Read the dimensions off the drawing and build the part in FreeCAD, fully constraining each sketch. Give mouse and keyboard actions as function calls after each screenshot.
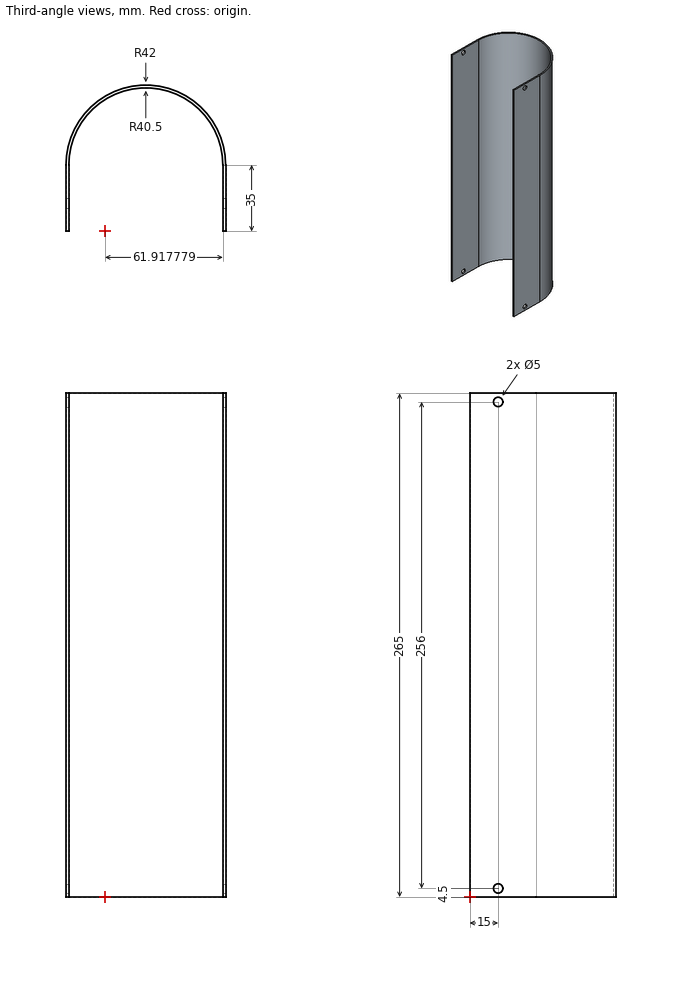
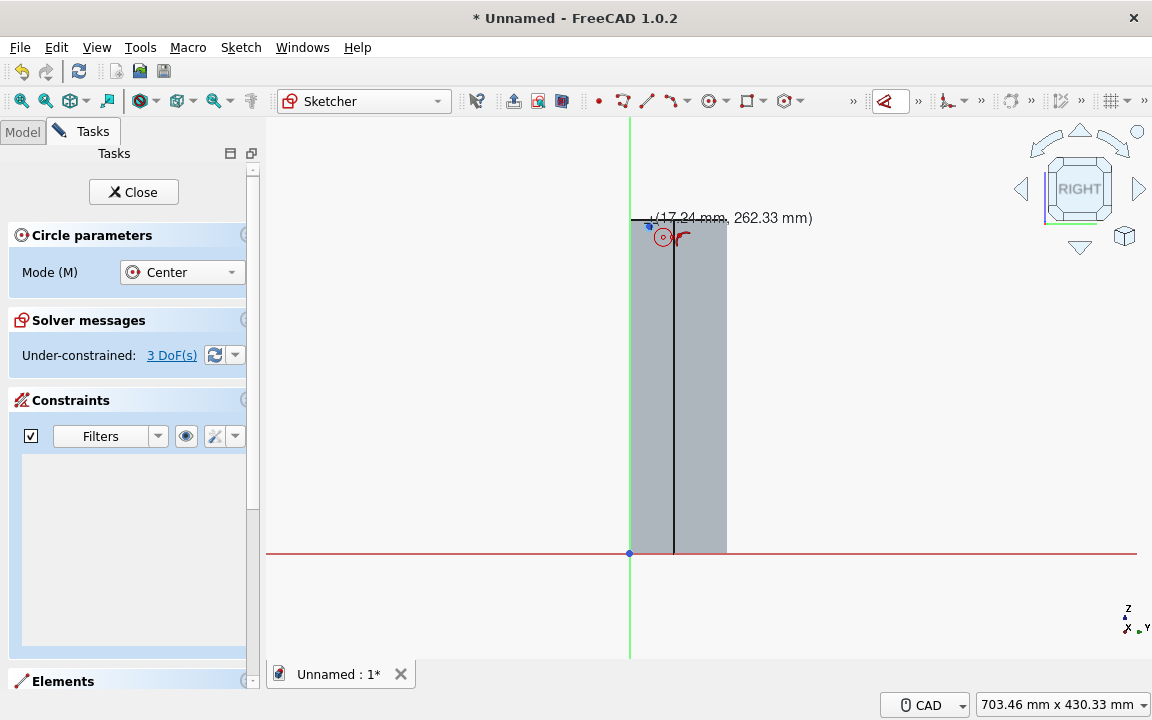
scroll(649, 548, up, 10)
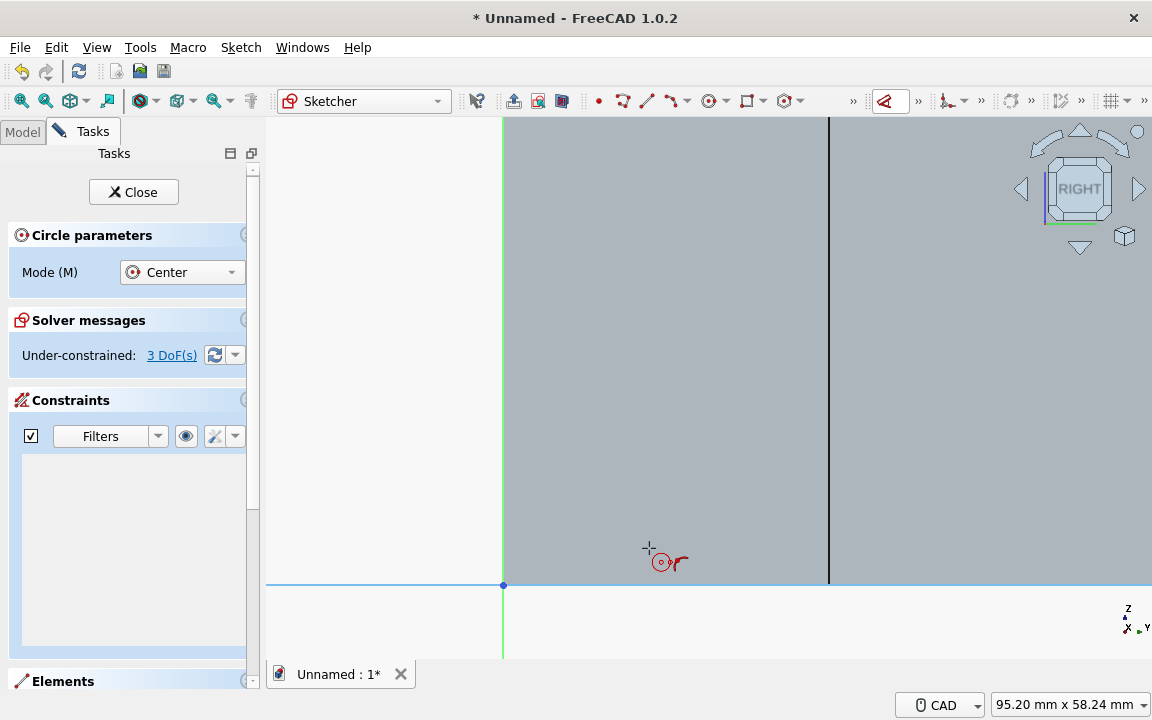
click(643, 543)
click(659, 527)
key(Escape)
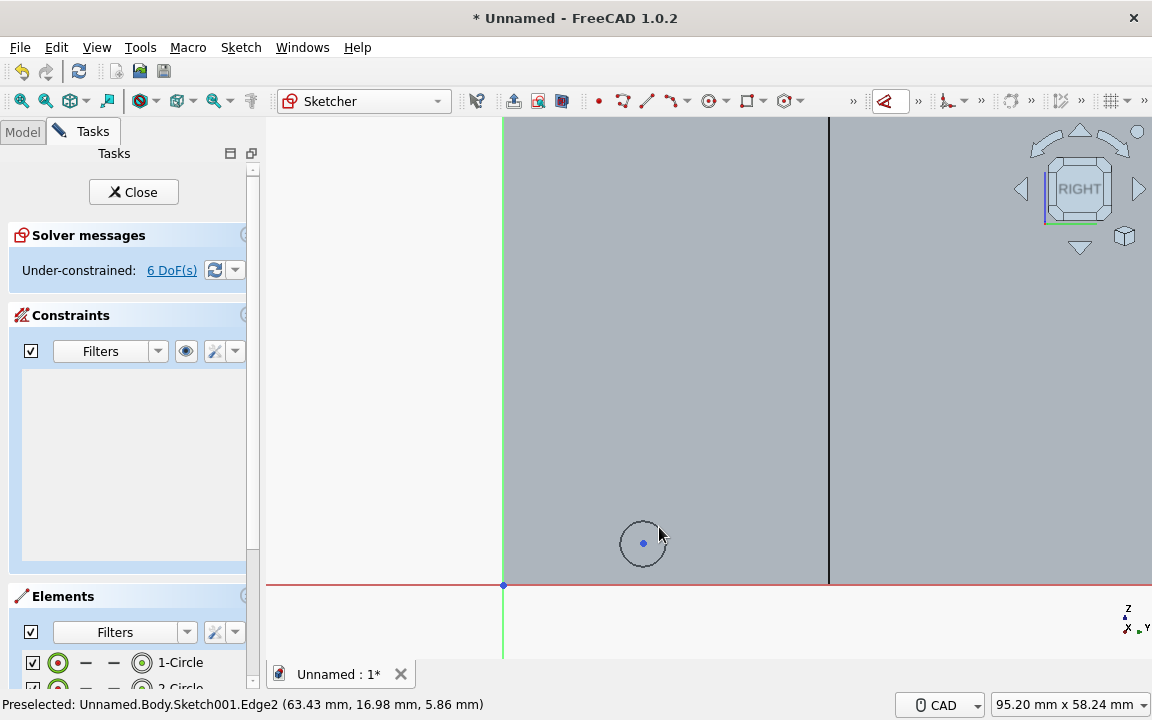
scroll(649, 549, down, 10)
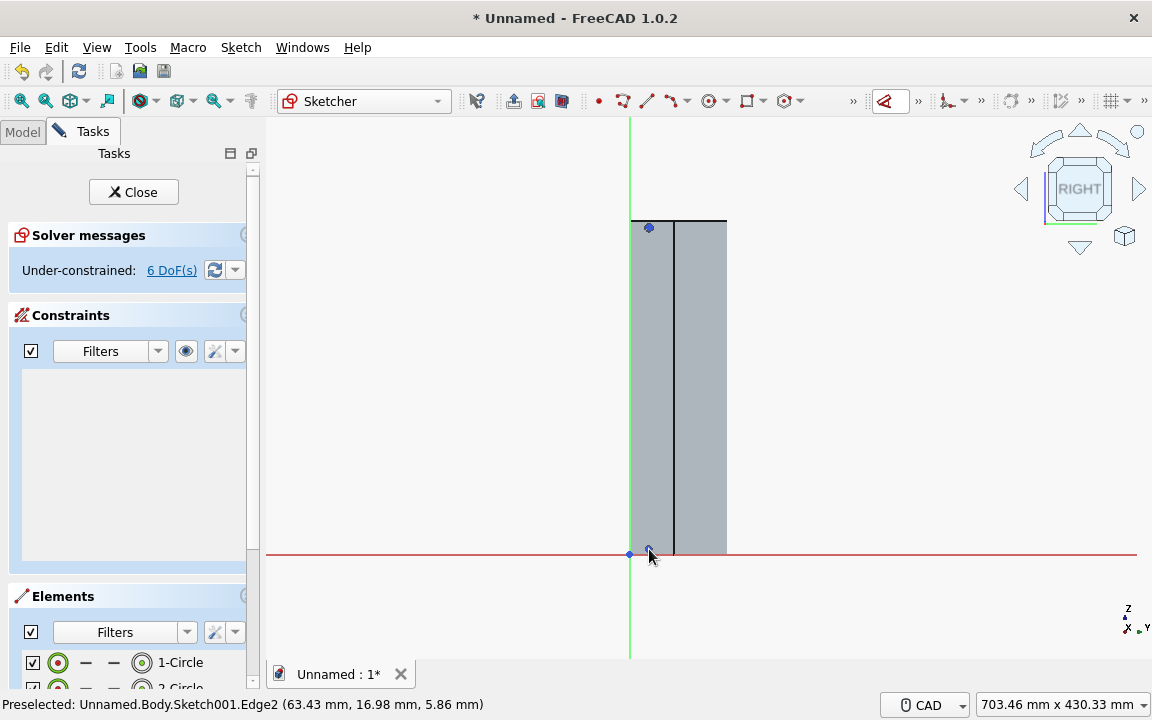
scroll(652, 225, up, 7)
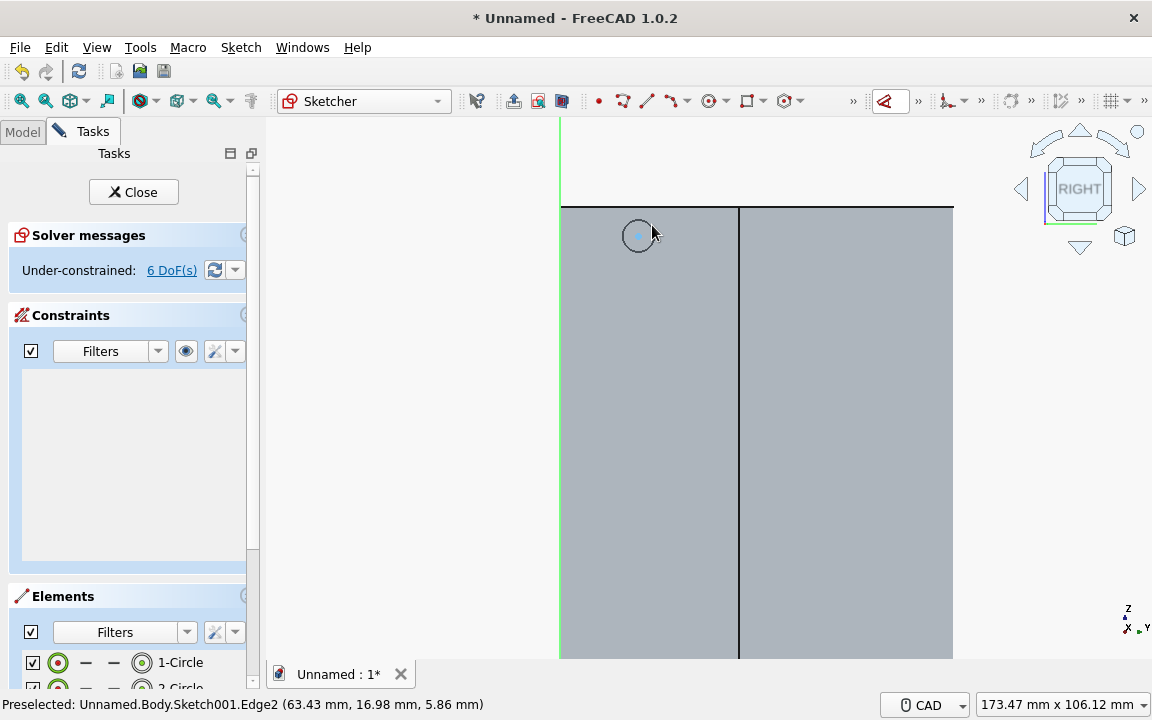
click(650, 225)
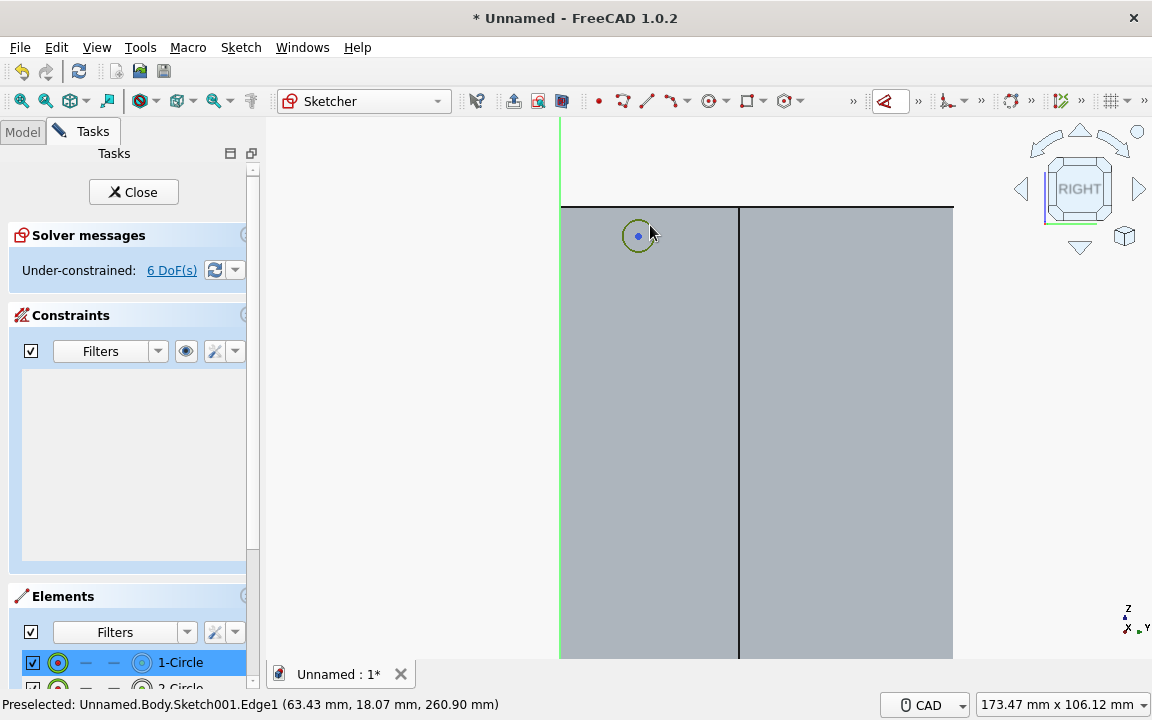
scroll(652, 224, down, 7)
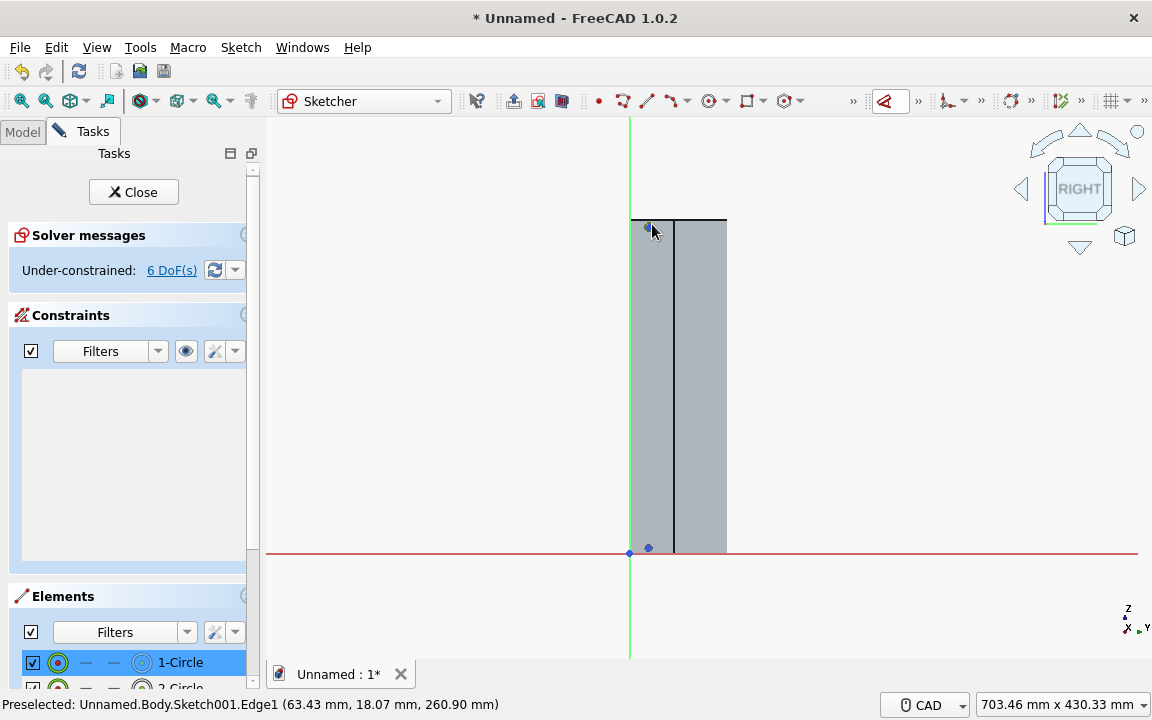
scroll(651, 546, up, 8)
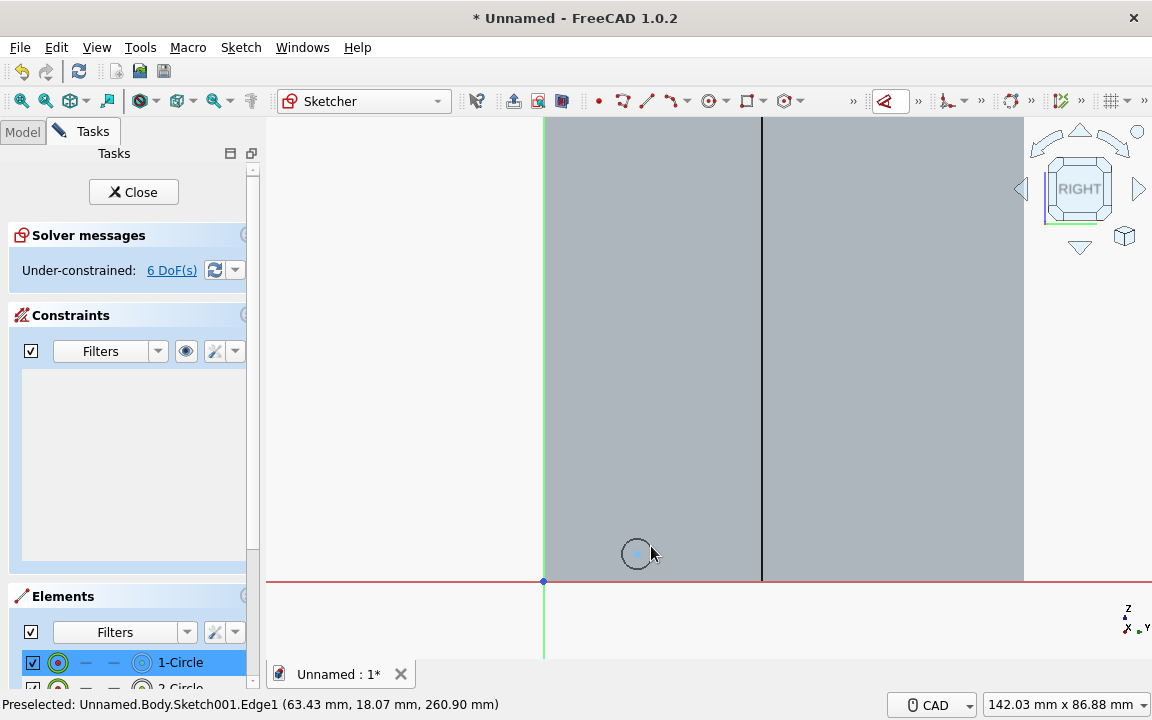
click(648, 543)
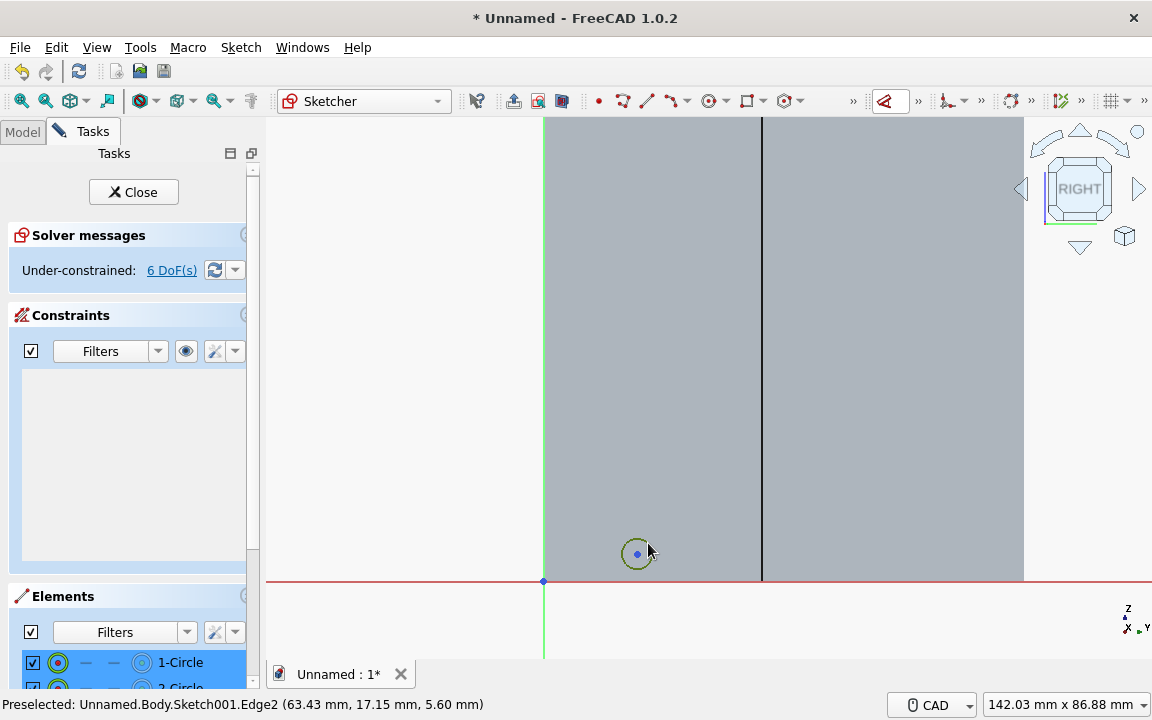
key(e)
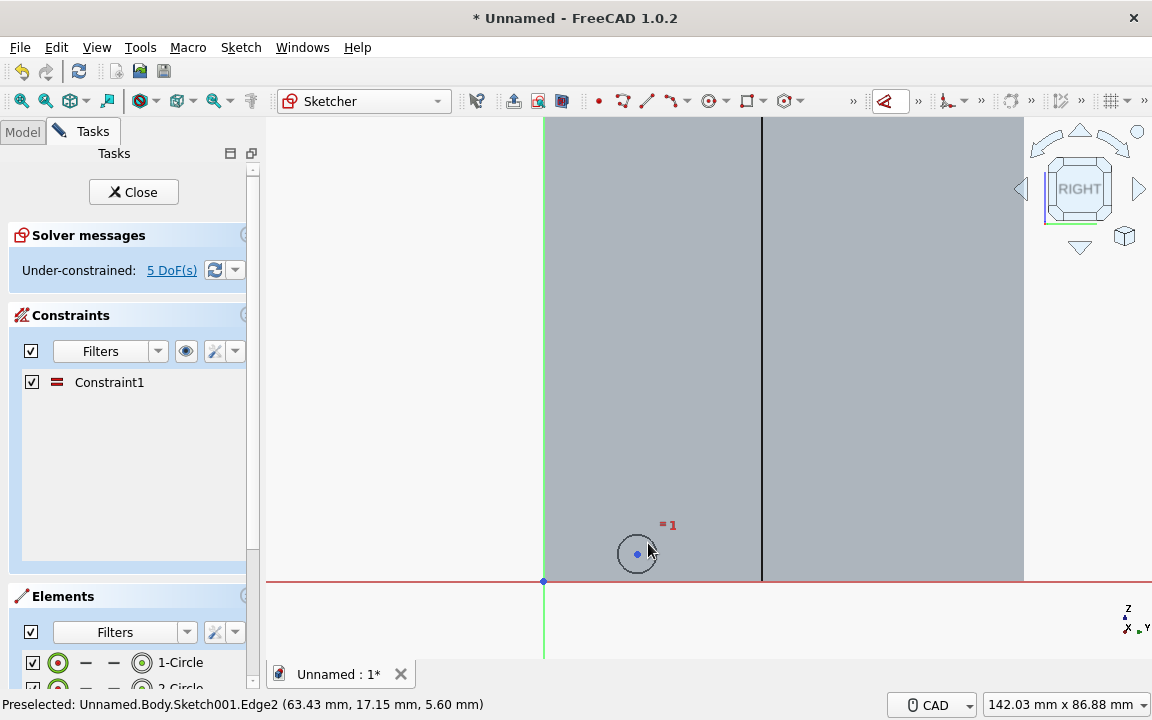
scroll(651, 547, down, 8)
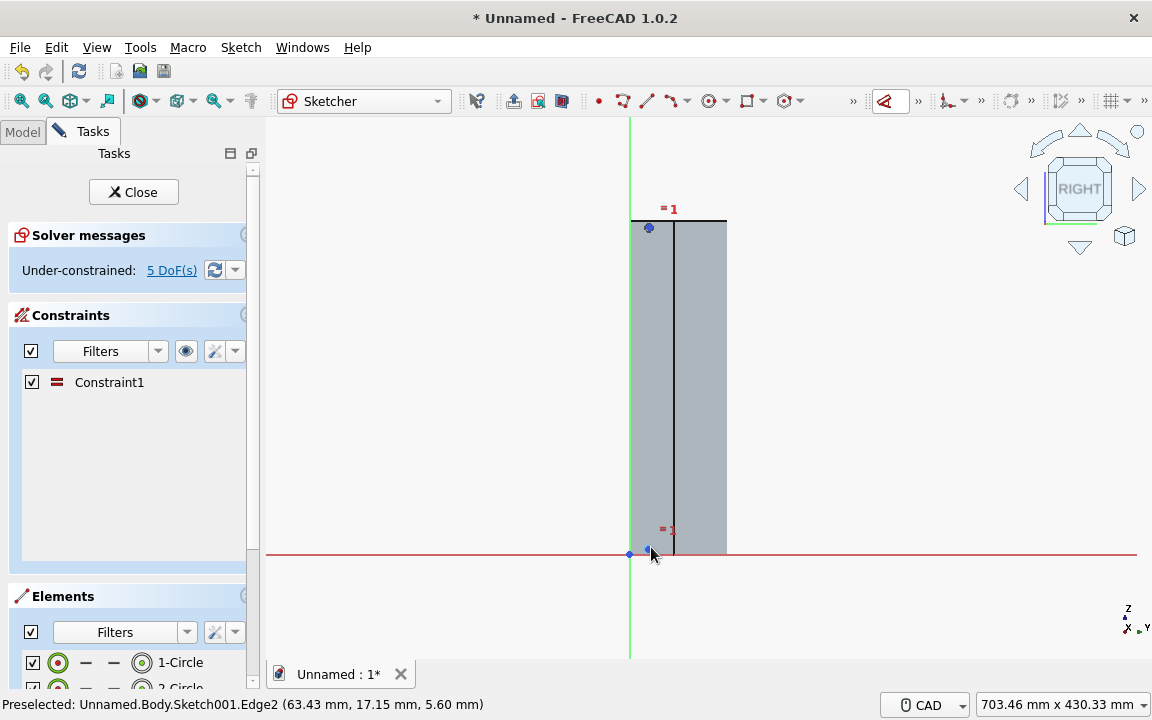
click(649, 228)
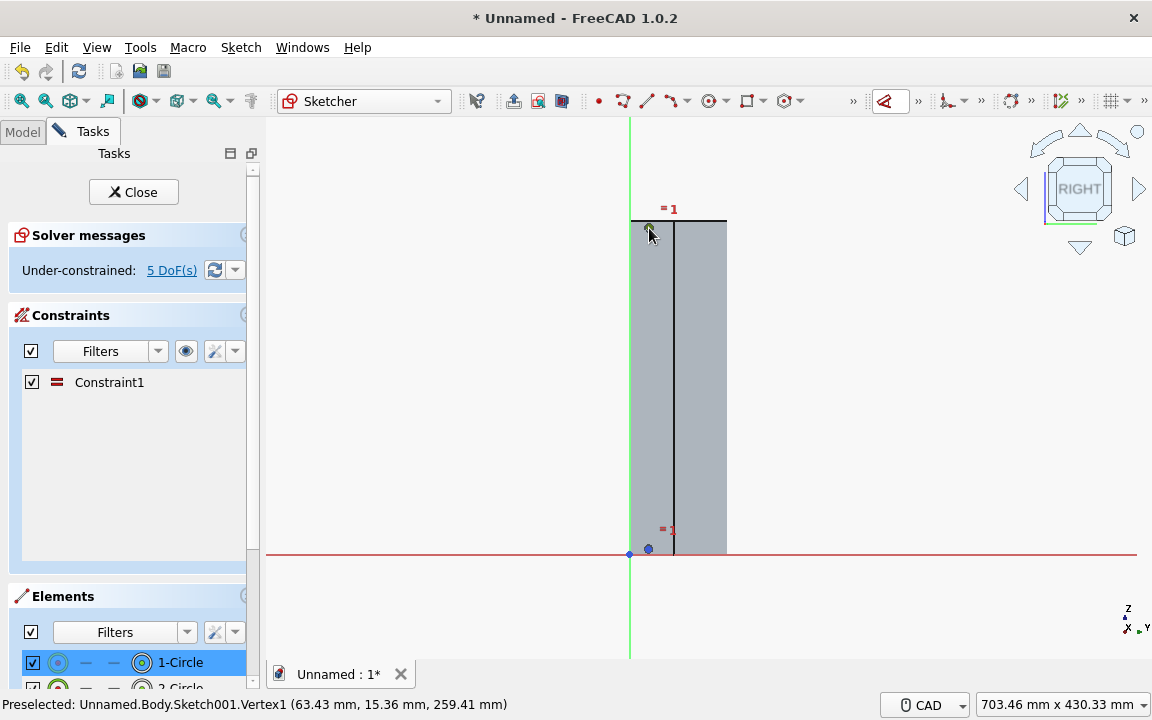
click(649, 549)